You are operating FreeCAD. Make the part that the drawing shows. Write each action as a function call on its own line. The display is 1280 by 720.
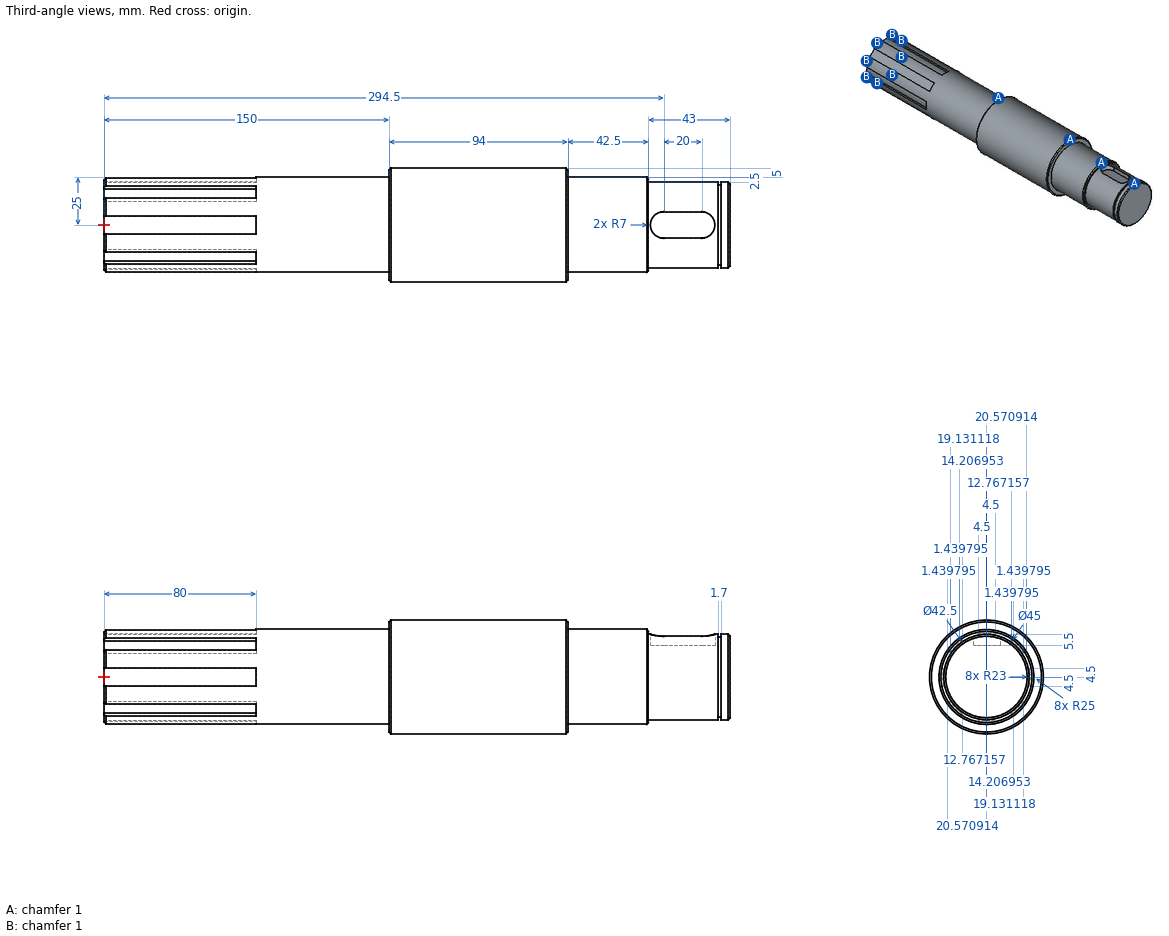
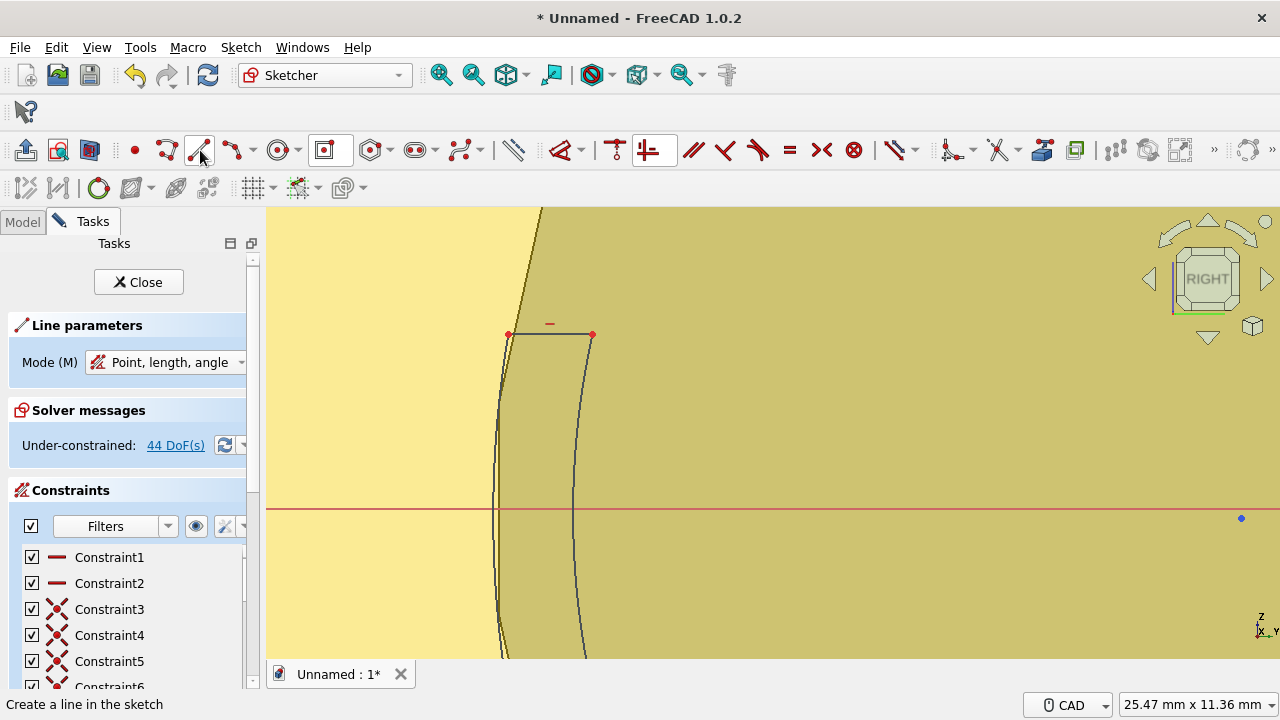
scroll(582, 421, down, 10)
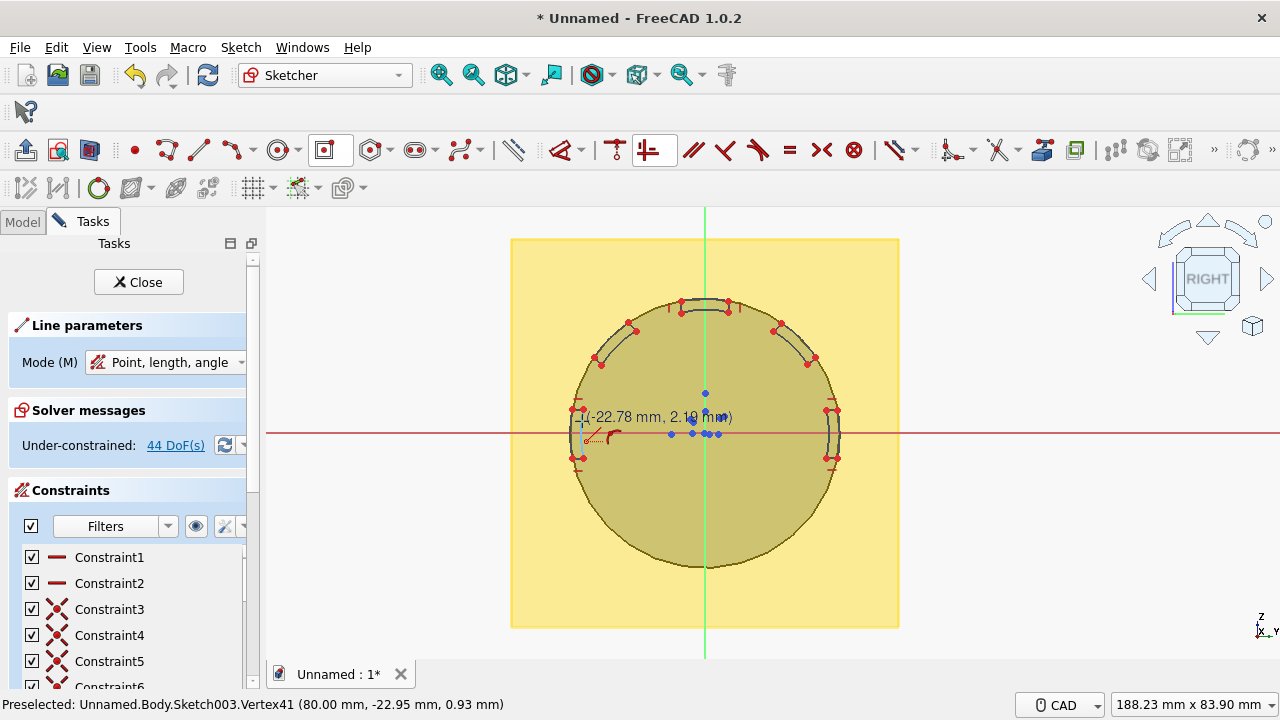
click(636, 536)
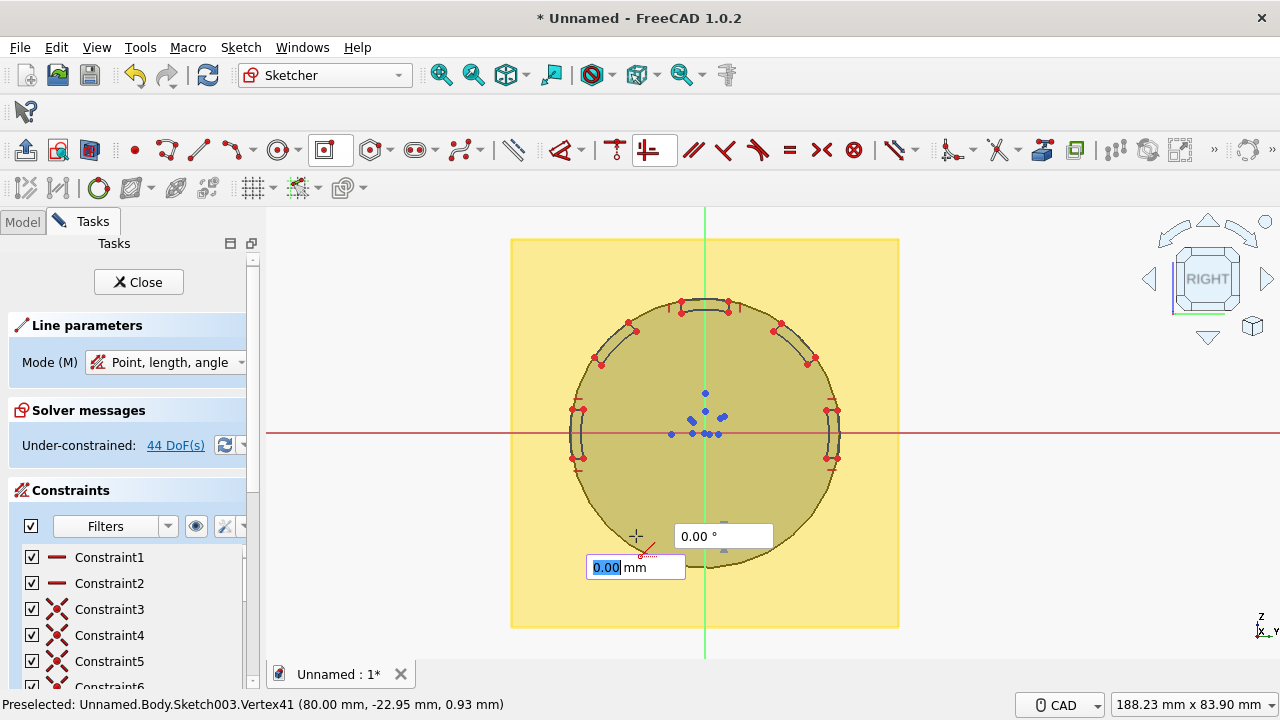
scroll(628, 544, up, 2)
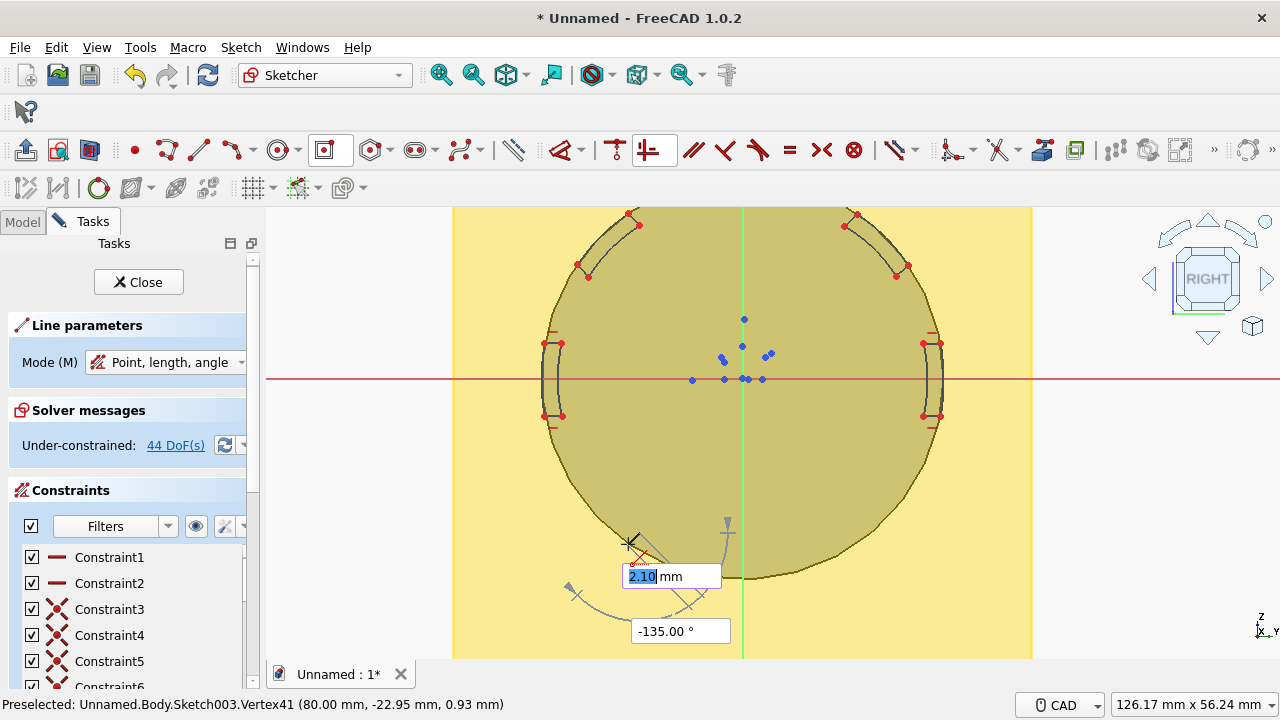
click(628, 544)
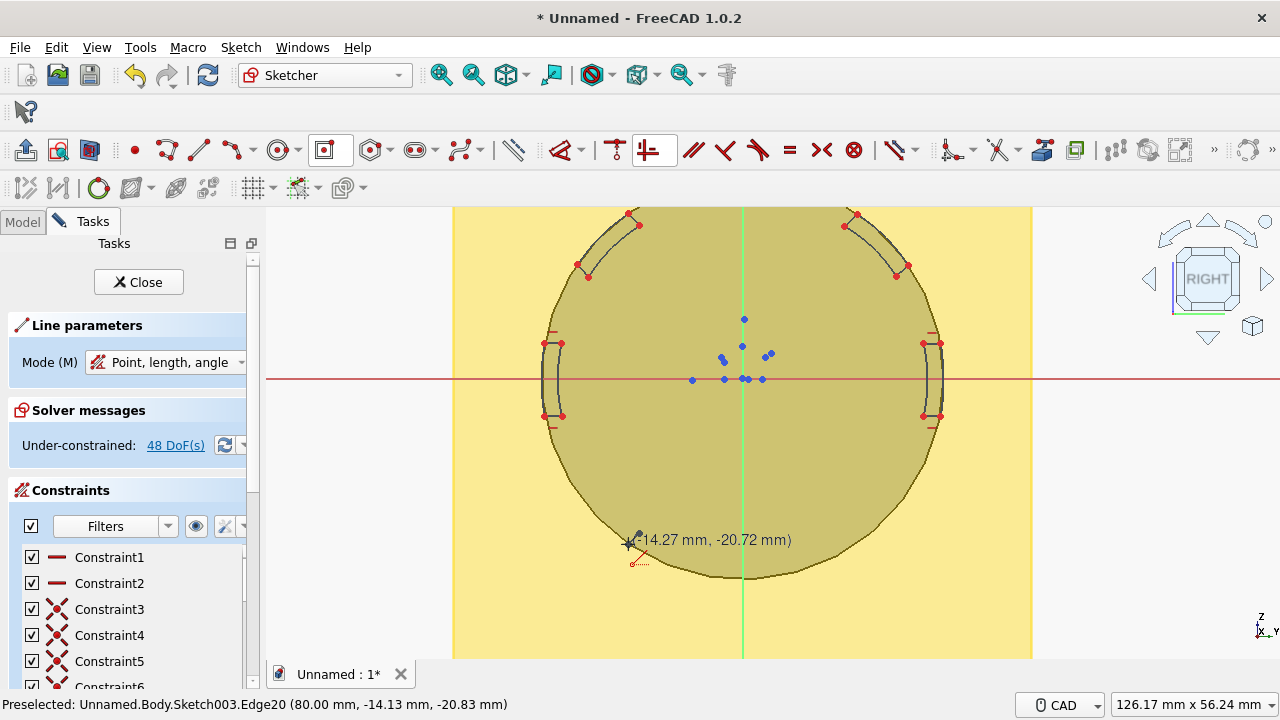
click(577, 493)
click(589, 481)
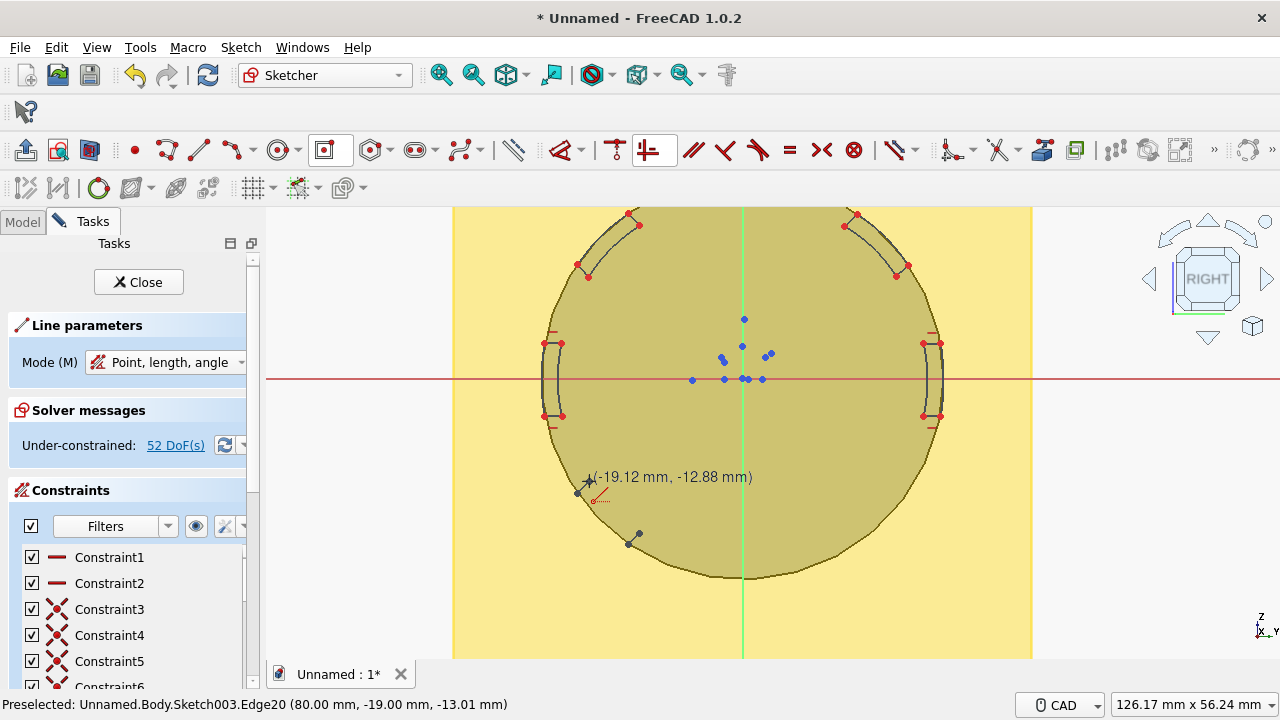
click(232, 150)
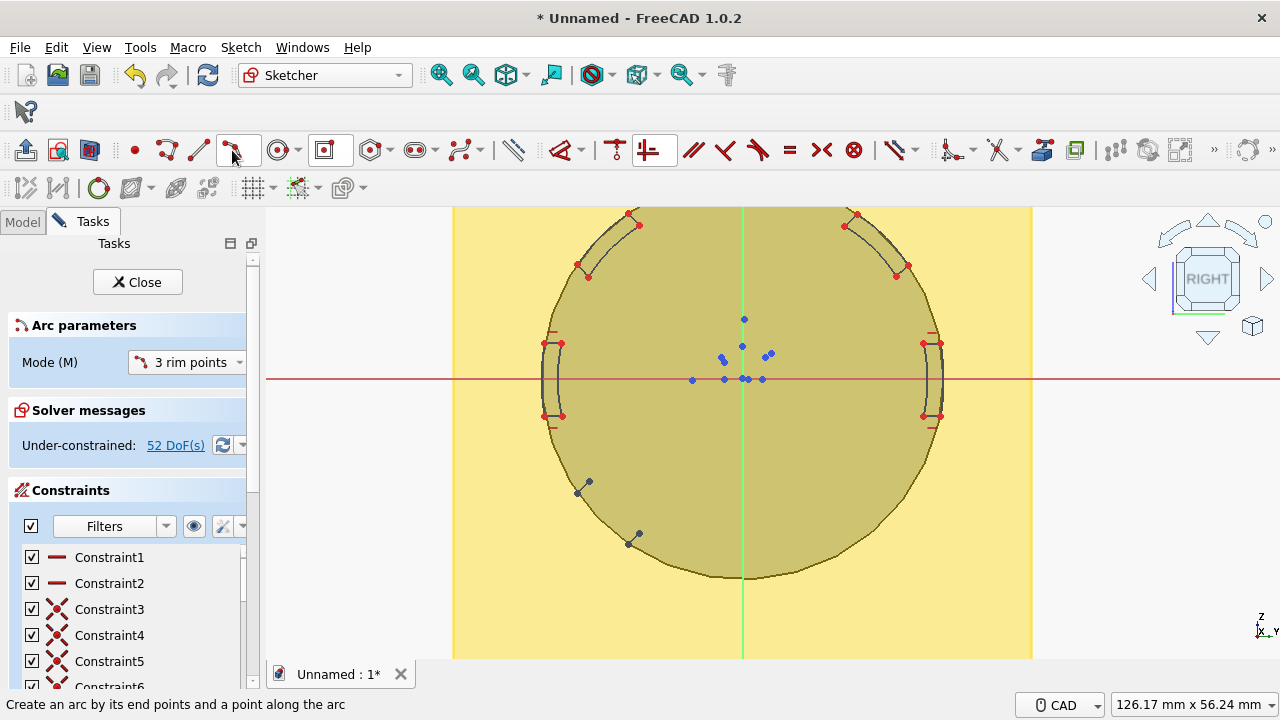
scroll(628, 544, up, 4)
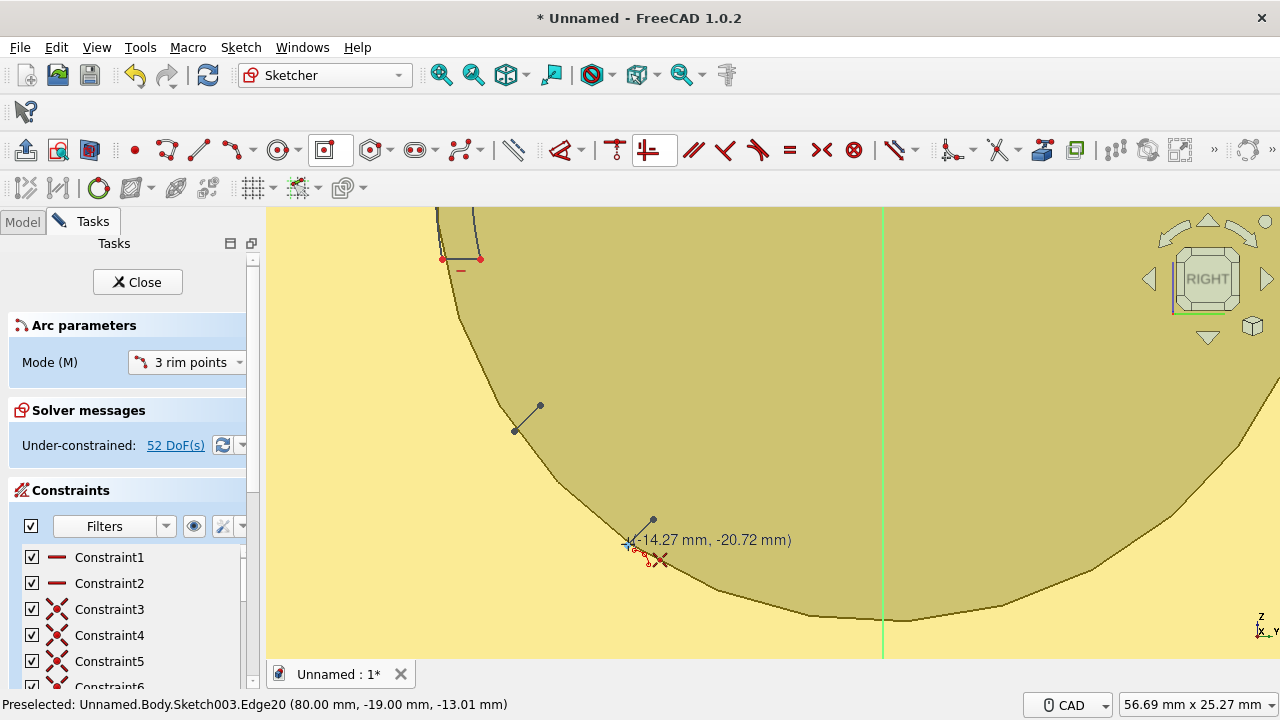
click(628, 545)
click(514, 432)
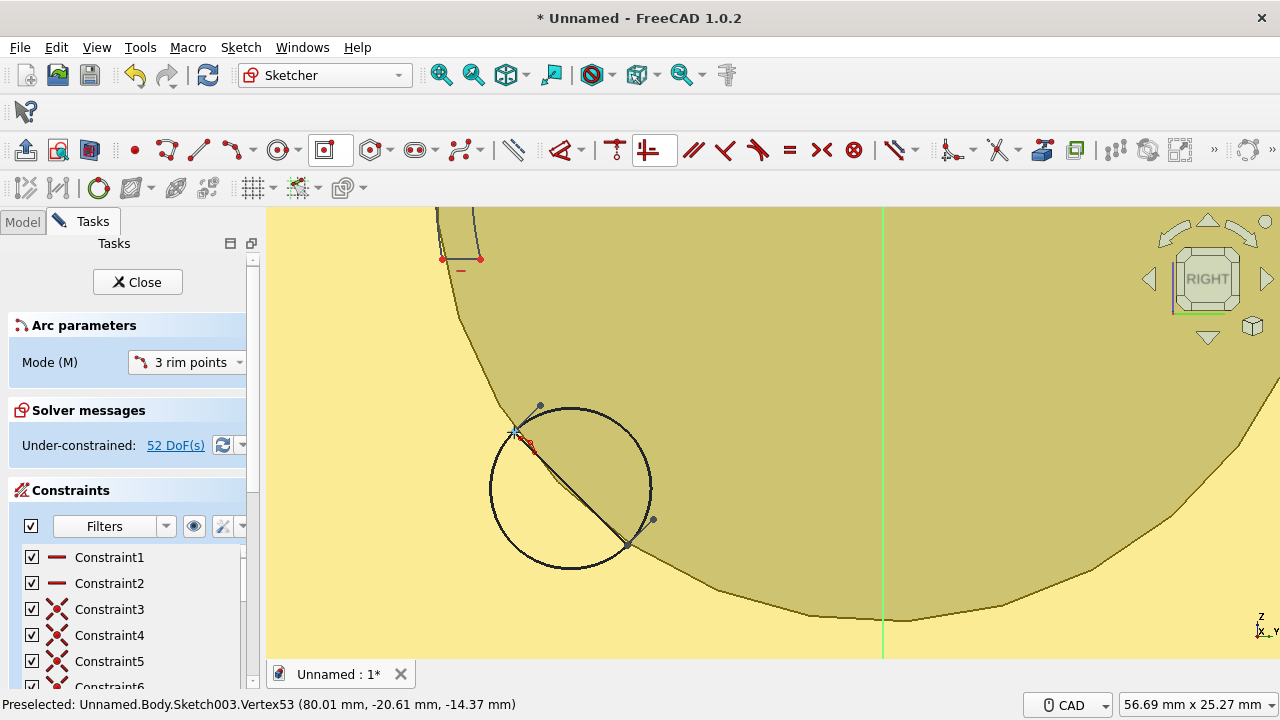
scroll(567, 491, up, 4)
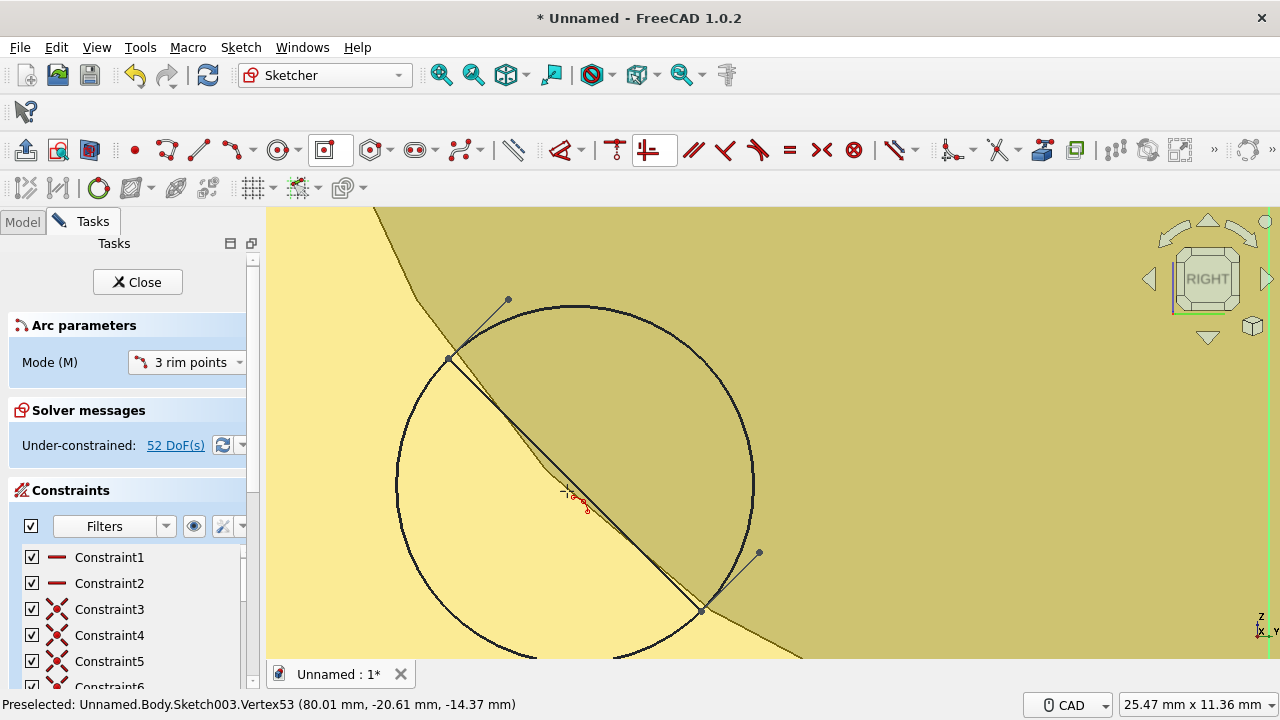
click(566, 490)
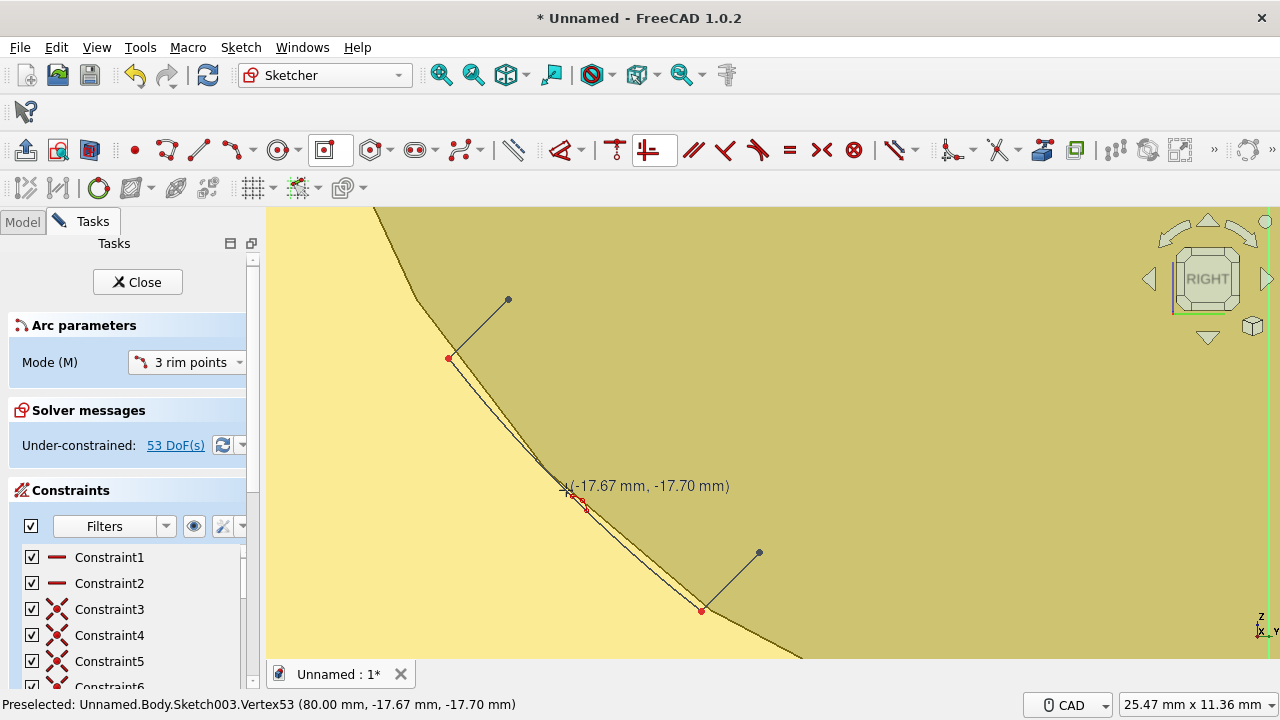
click(508, 299)
click(760, 553)
click(622, 434)